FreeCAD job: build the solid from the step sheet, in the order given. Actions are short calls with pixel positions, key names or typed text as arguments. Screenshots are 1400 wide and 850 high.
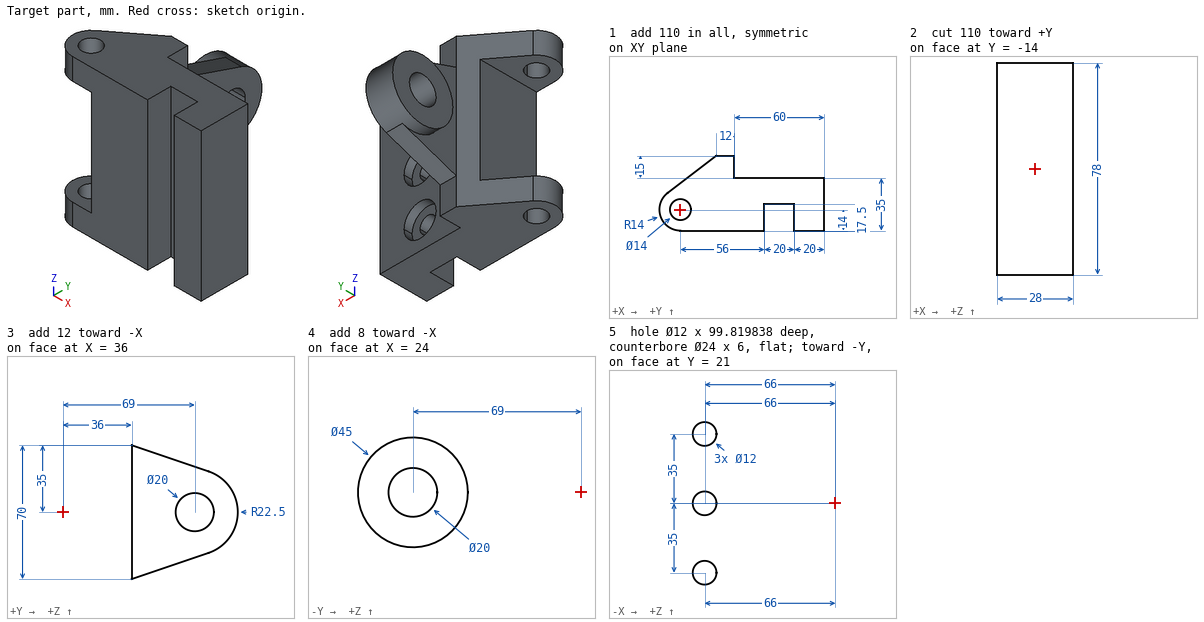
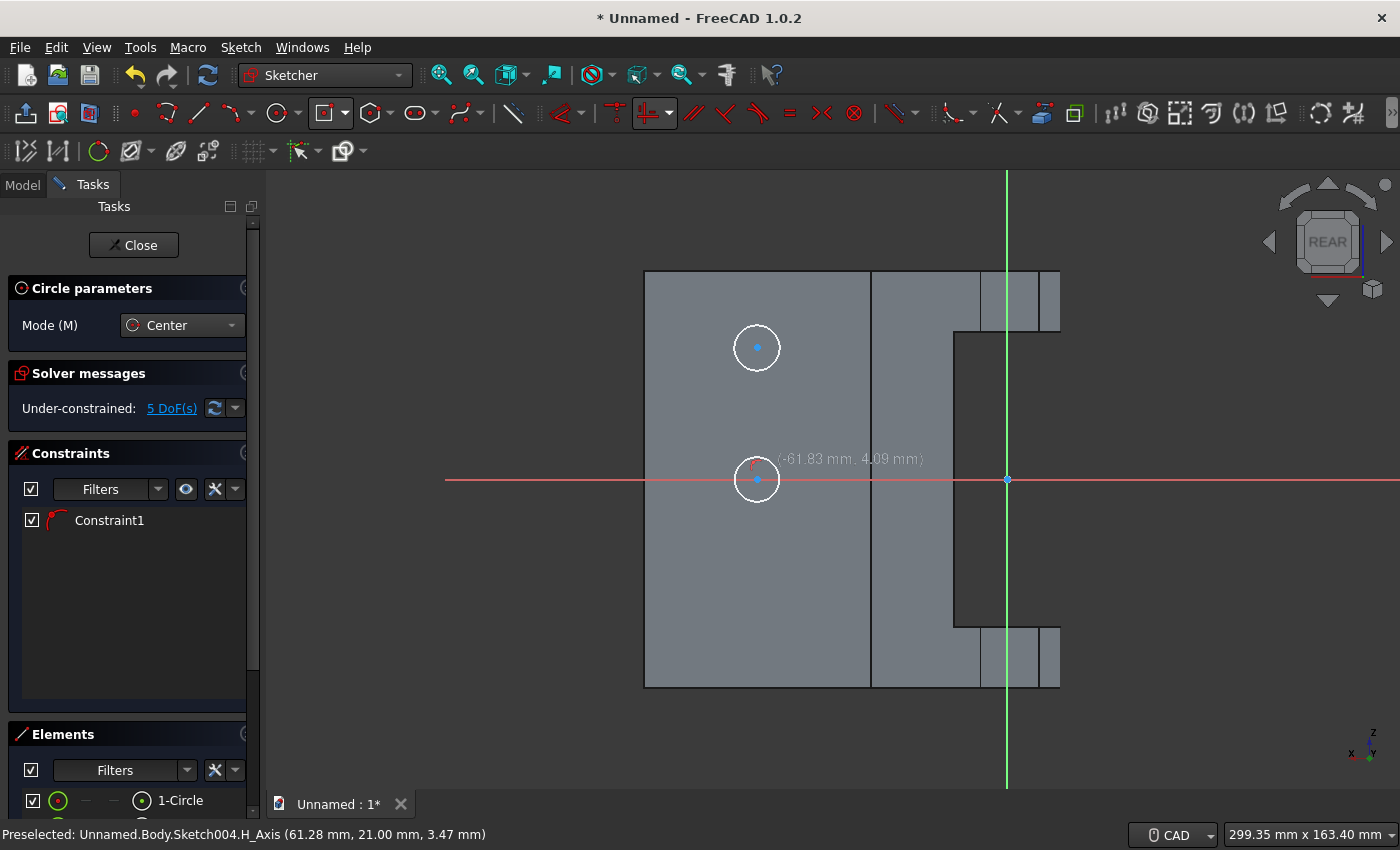
click(757, 612)
click(773, 596)
key(Escape)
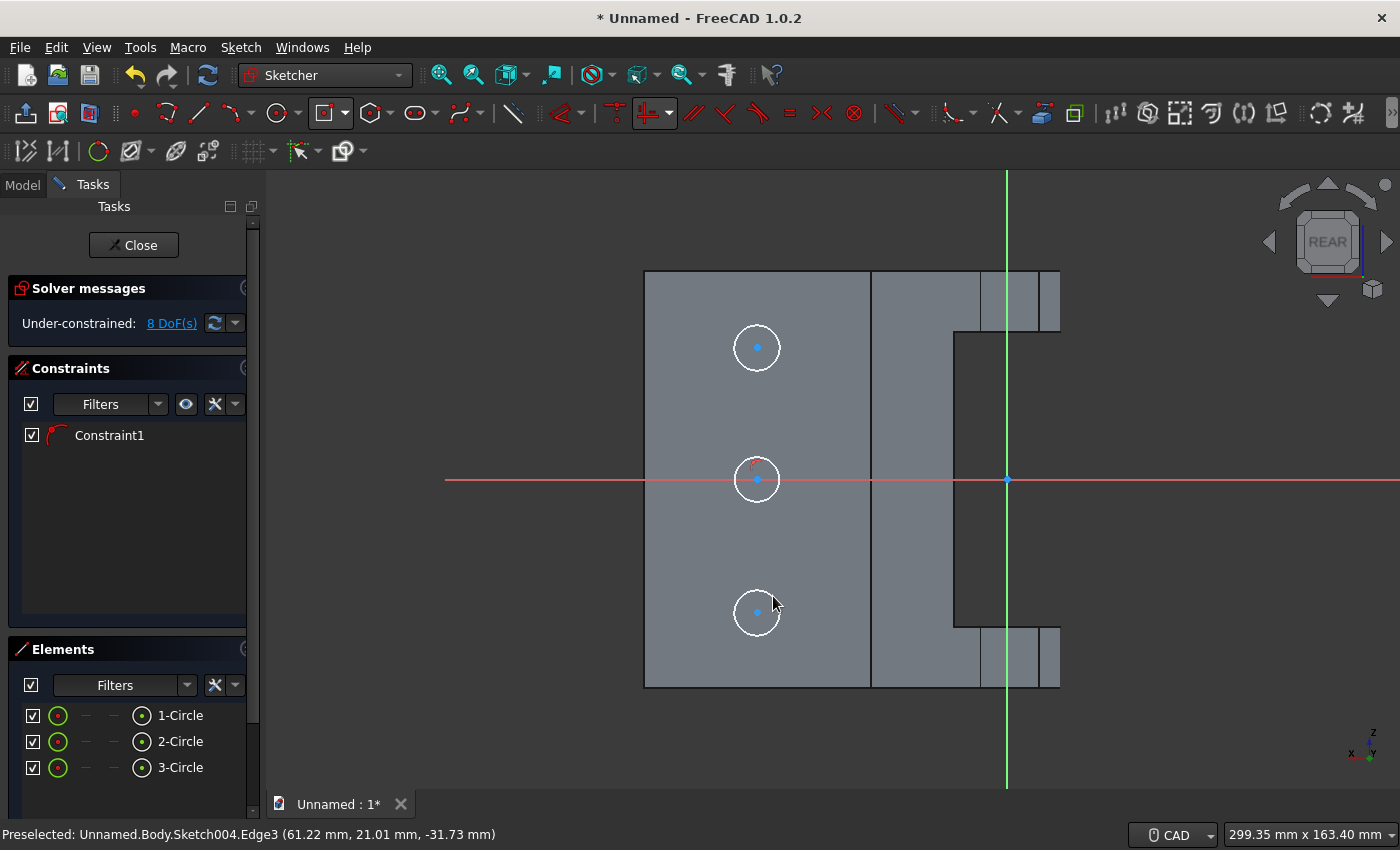
click(773, 332)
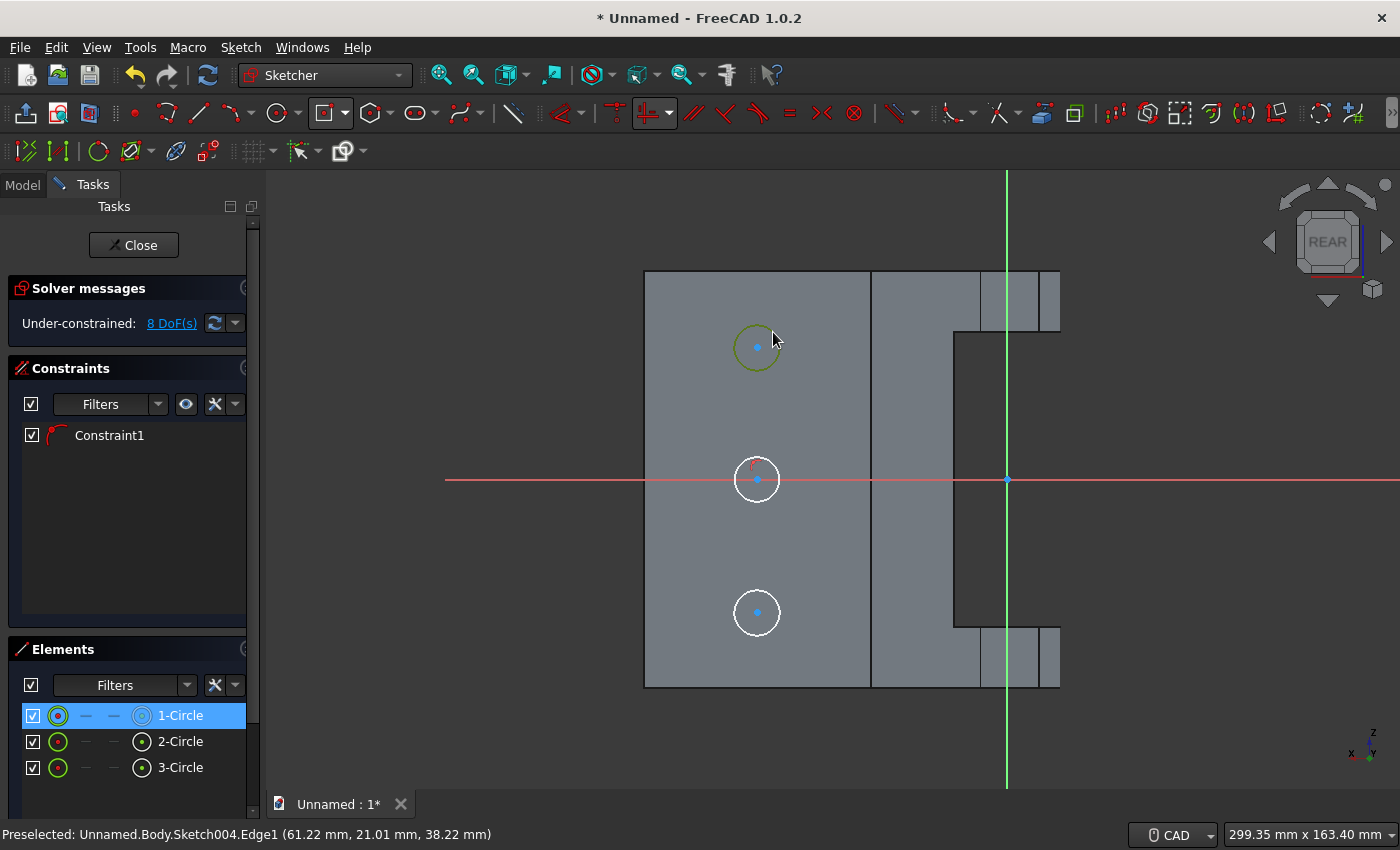
click(773, 464)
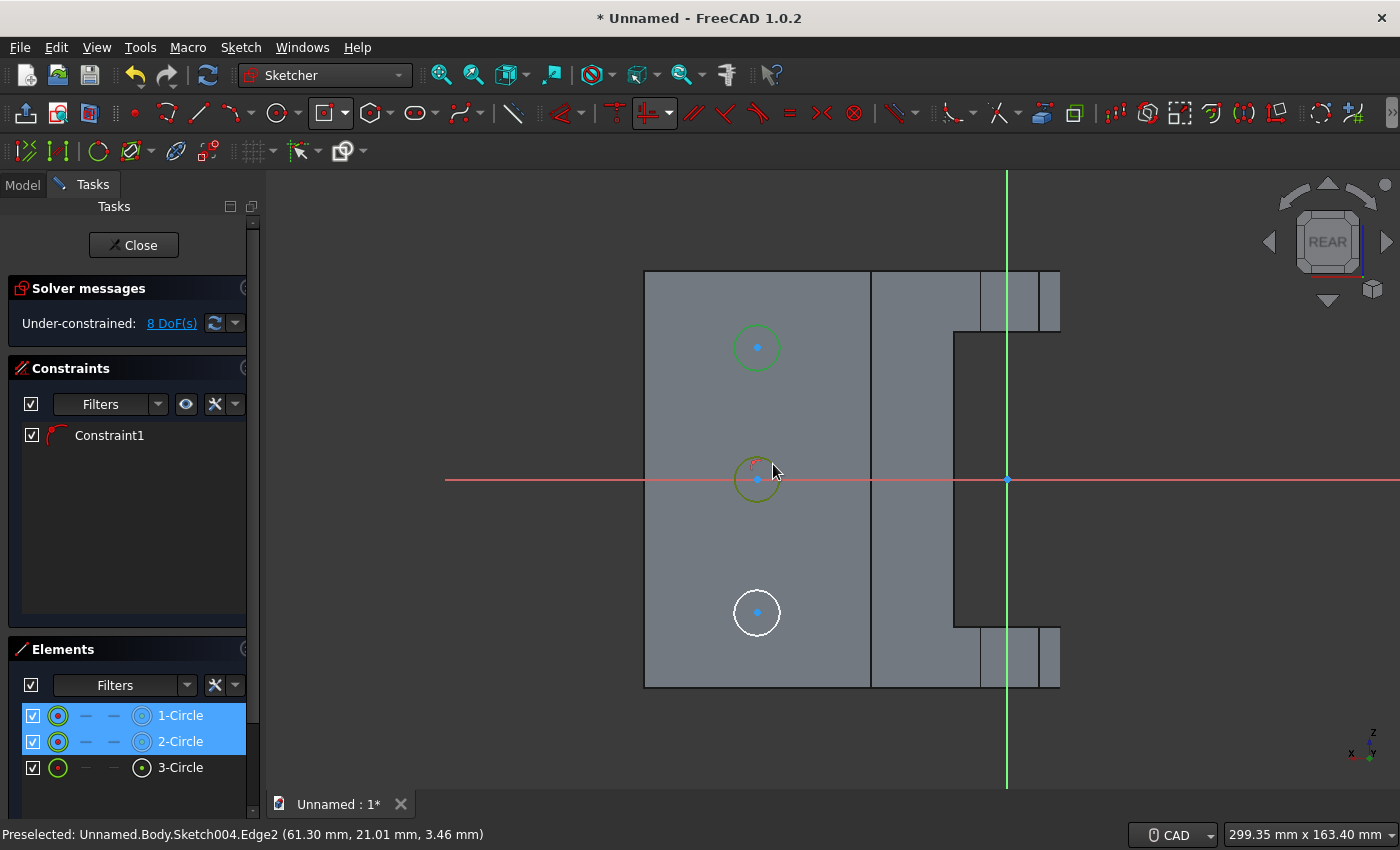
click(773, 597)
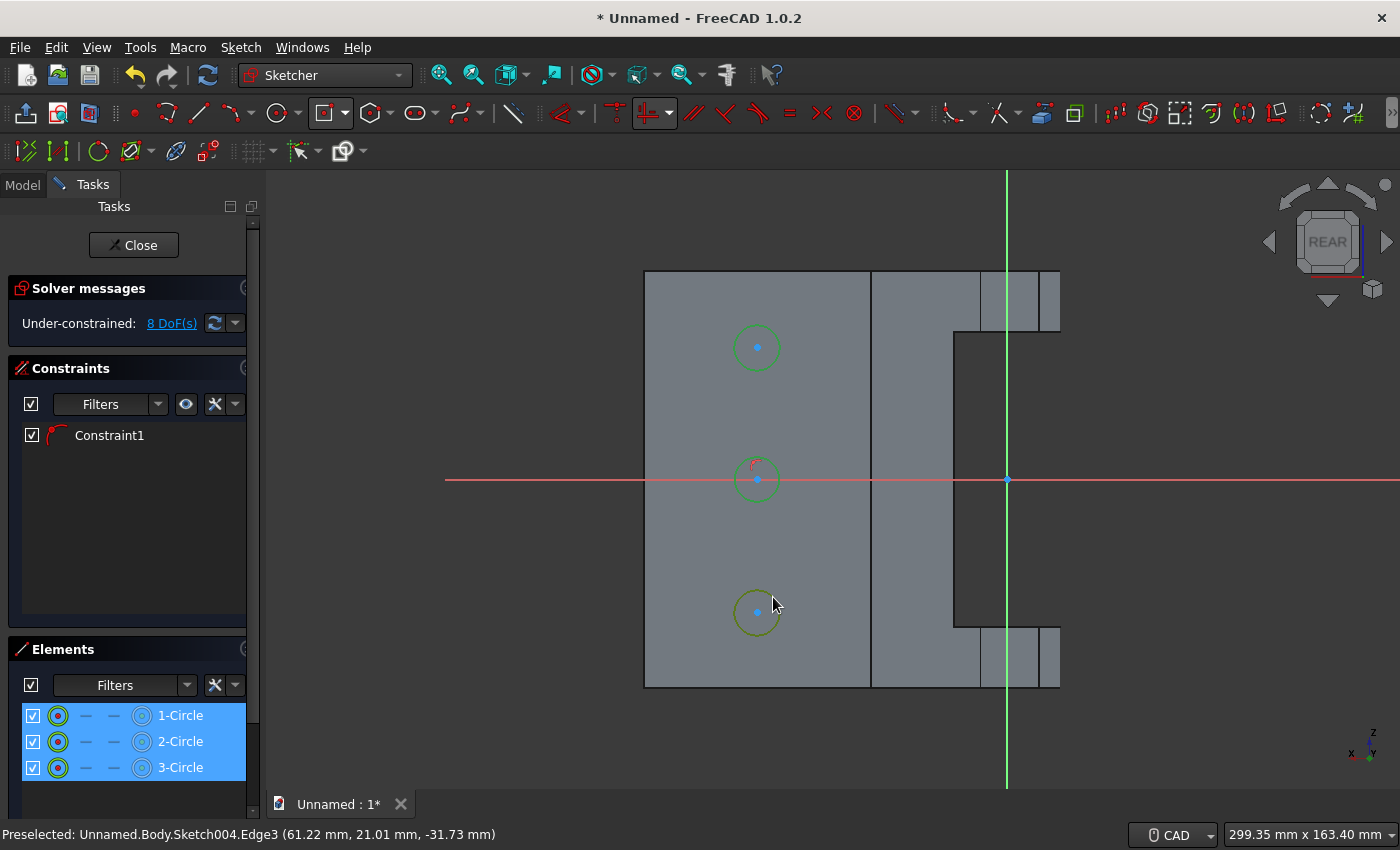
click(790, 114)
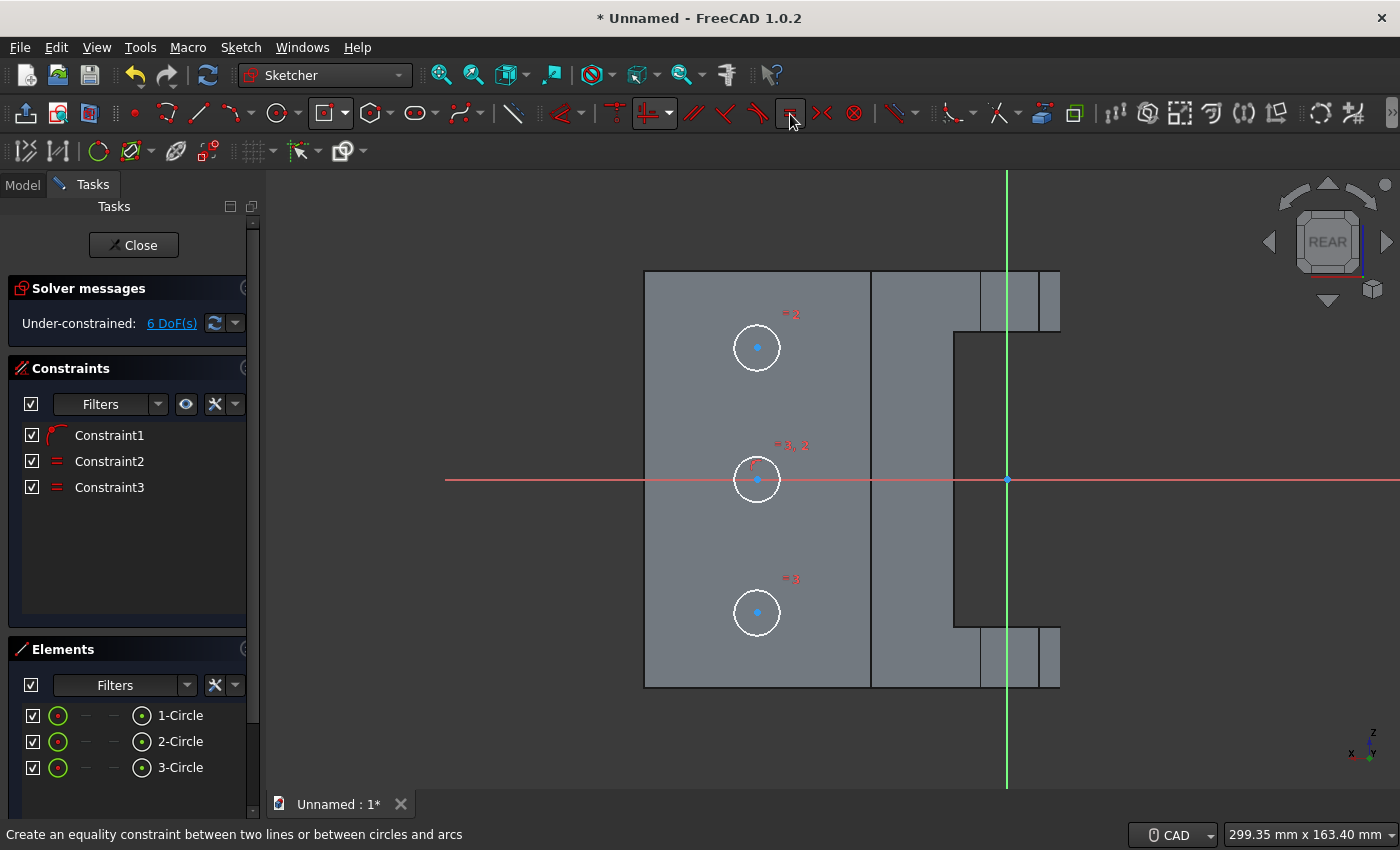
click(560, 114)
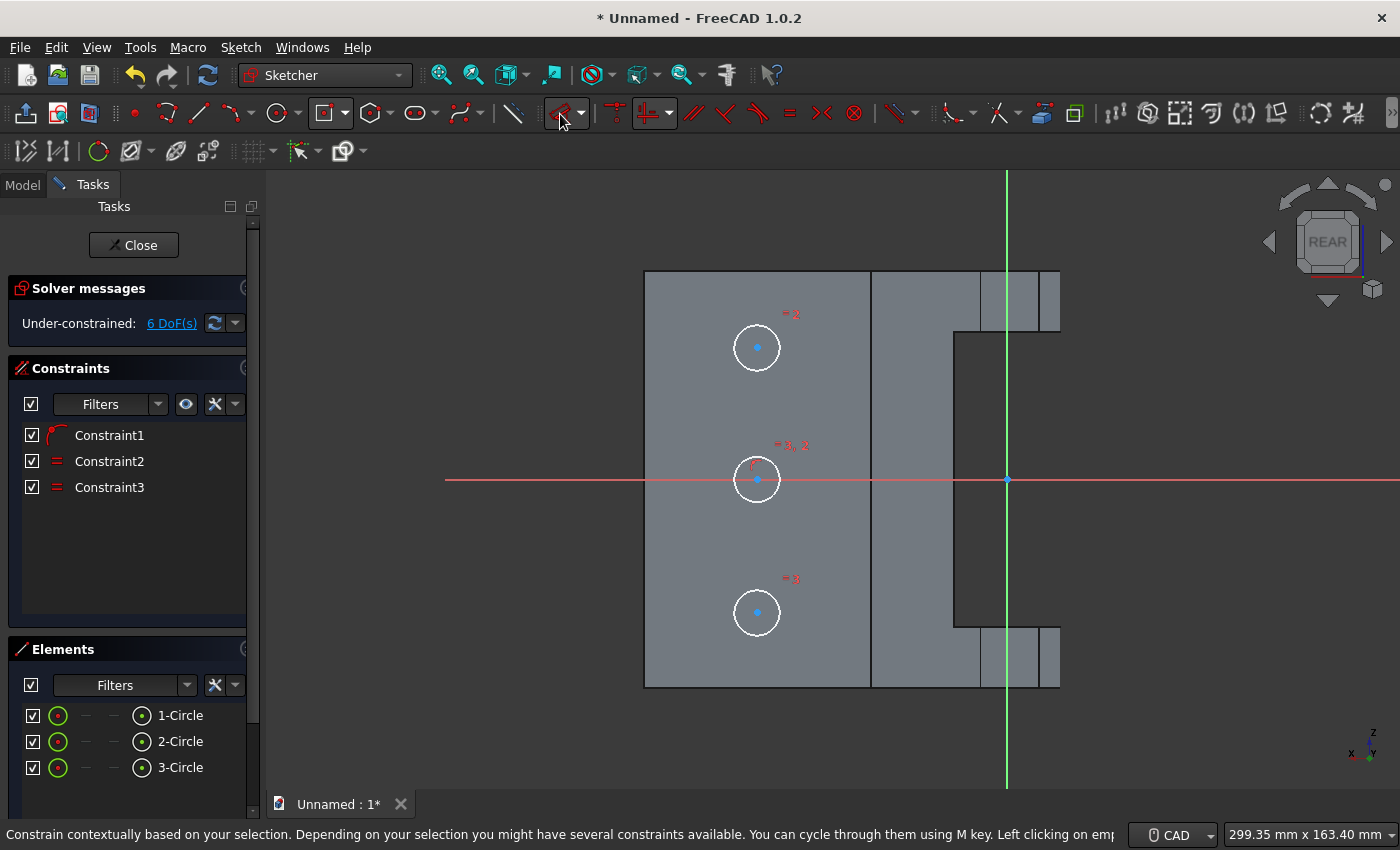
click(773, 332)
click(796, 309)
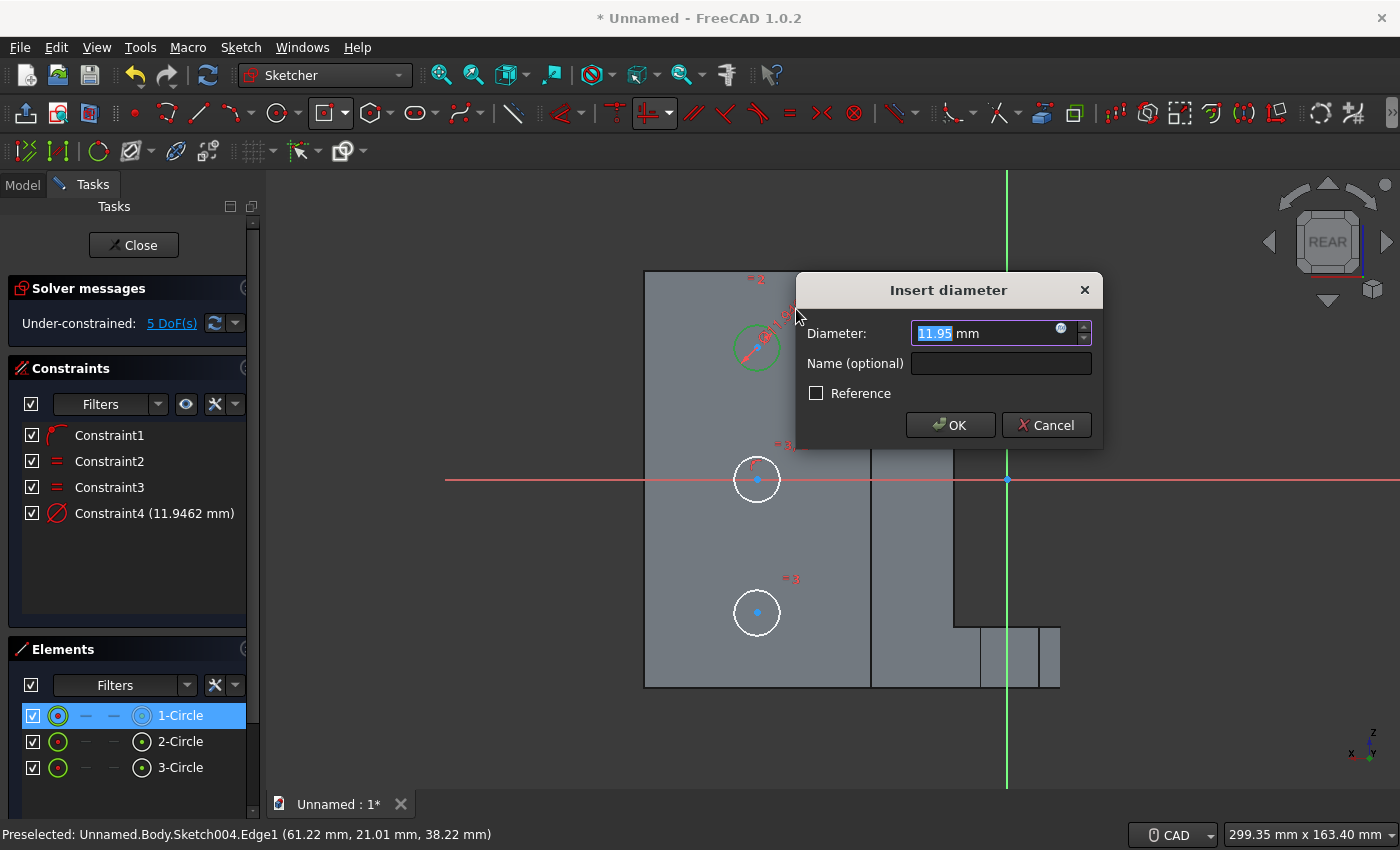
text(12)
key(Return)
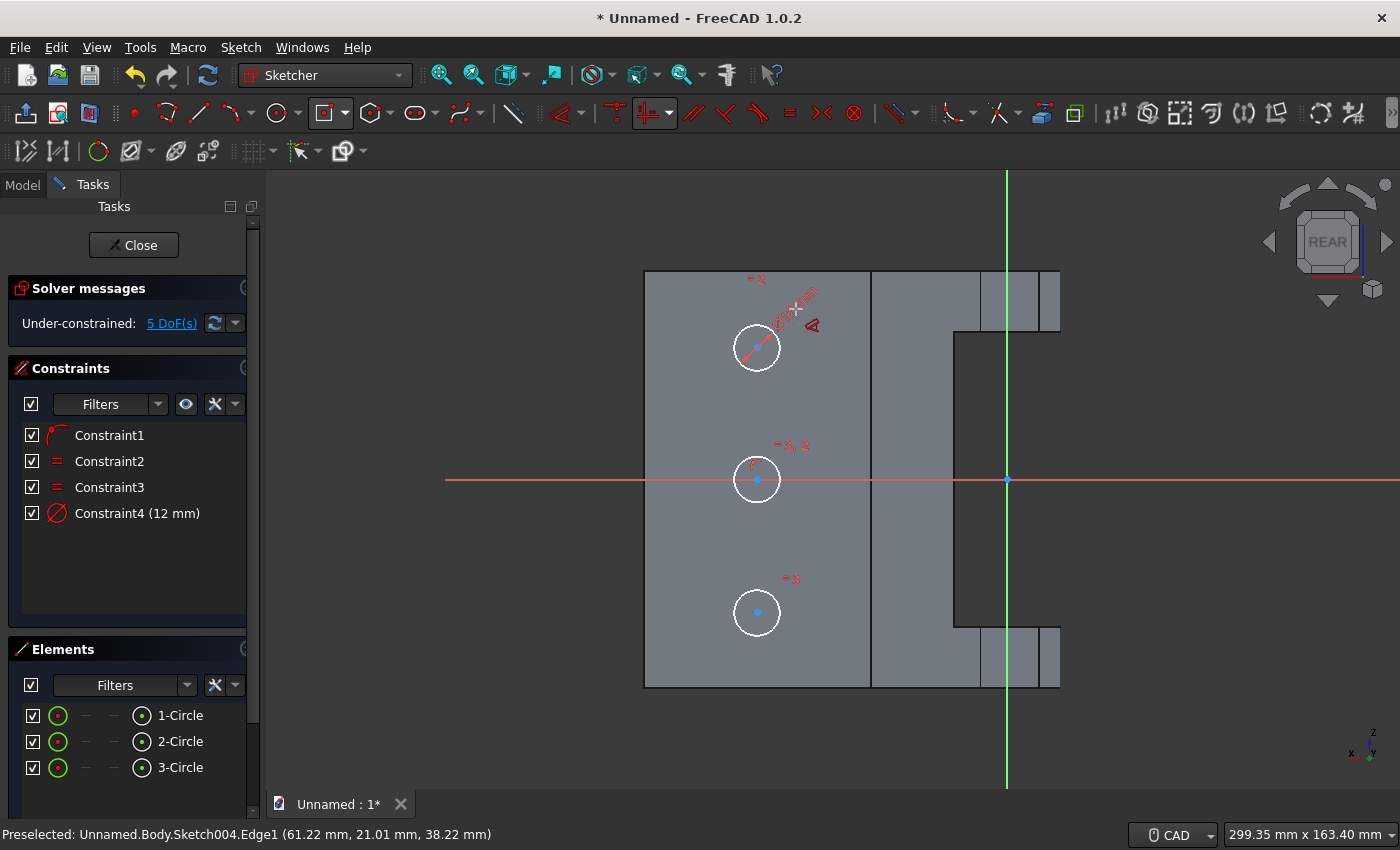
click(757, 348)
click(882, 314)